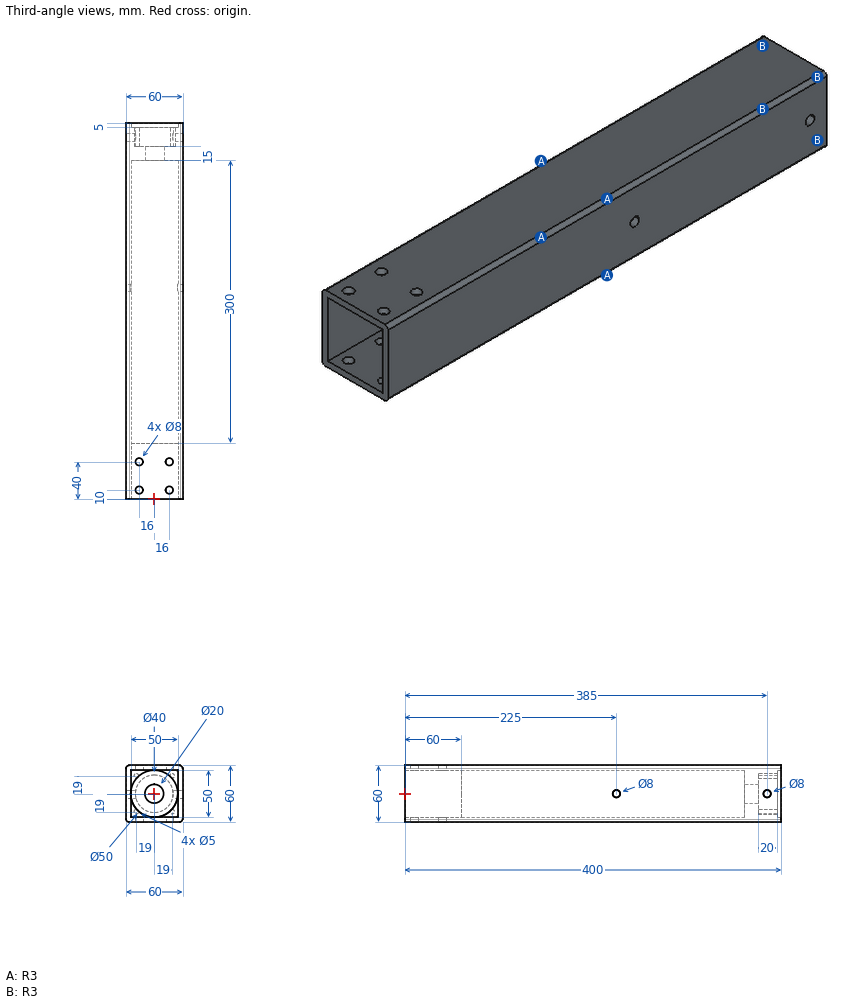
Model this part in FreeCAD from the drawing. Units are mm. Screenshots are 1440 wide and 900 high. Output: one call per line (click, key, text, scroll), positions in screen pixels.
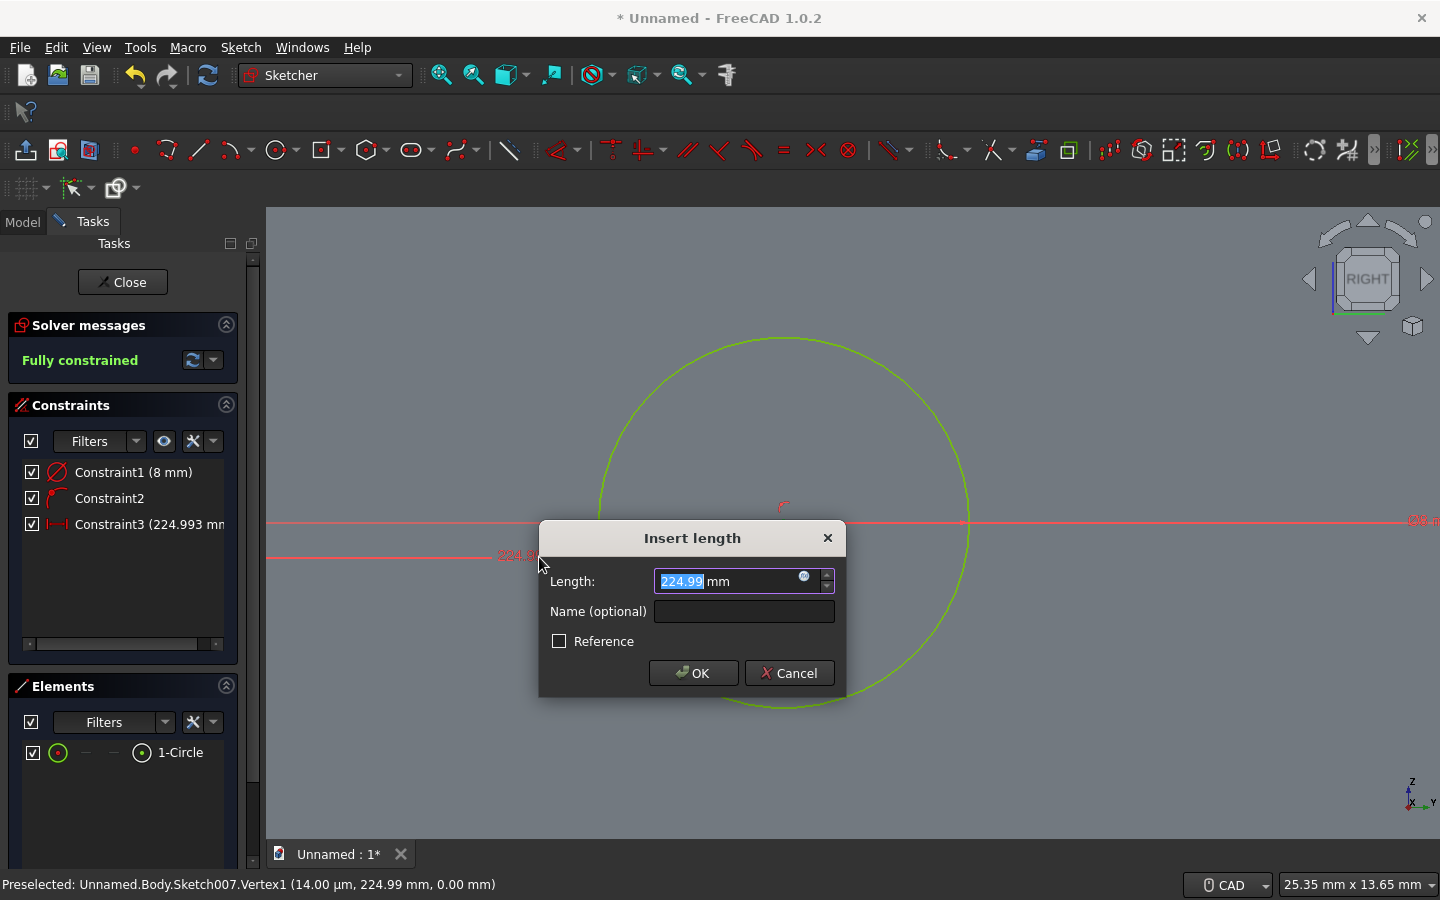
text(225)
key(Return)
key(Escape)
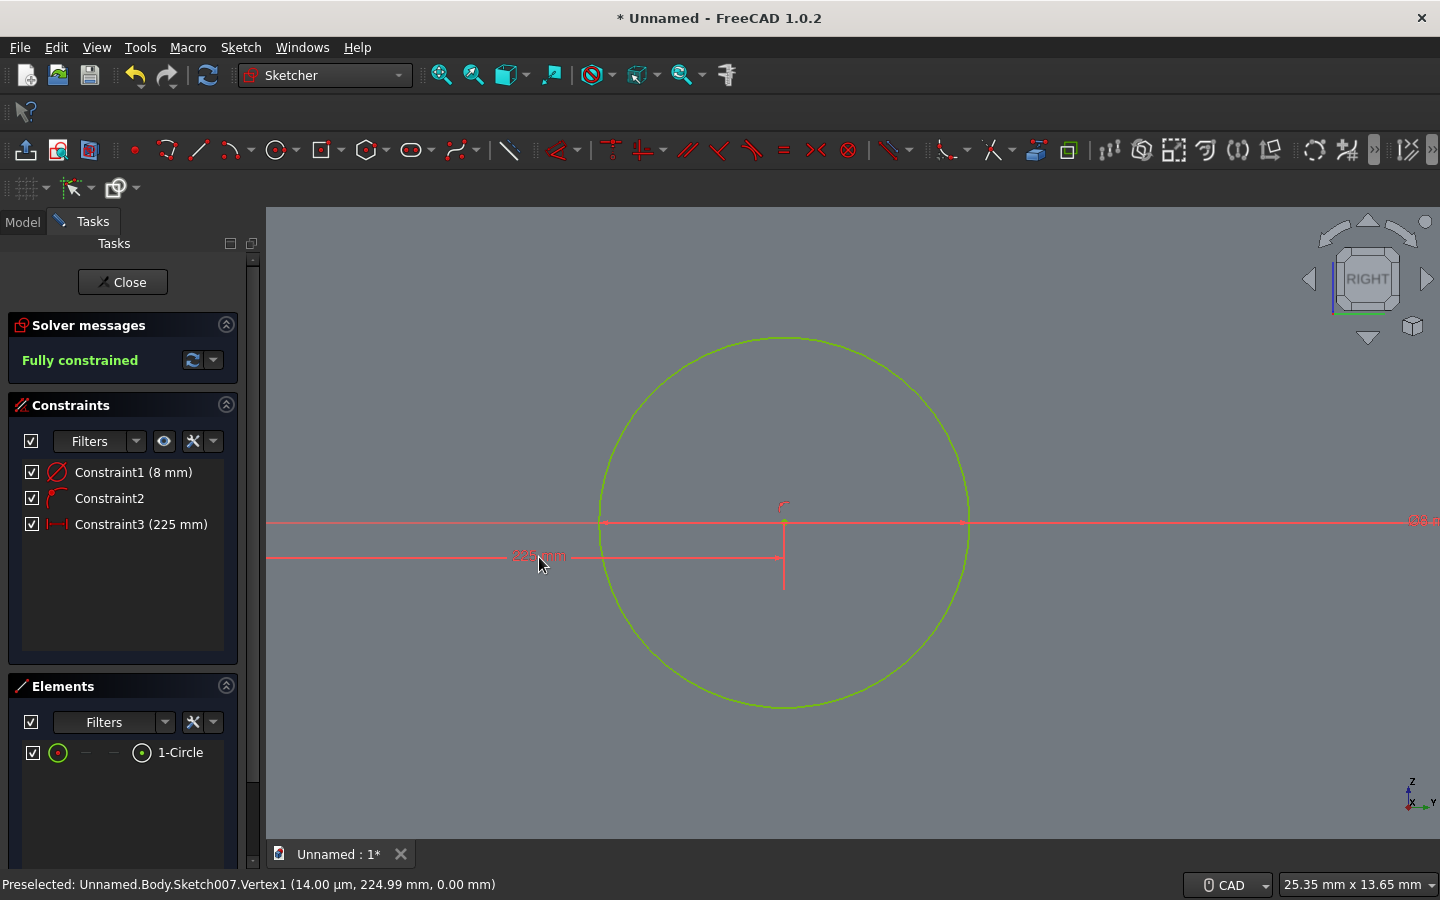
click(123, 282)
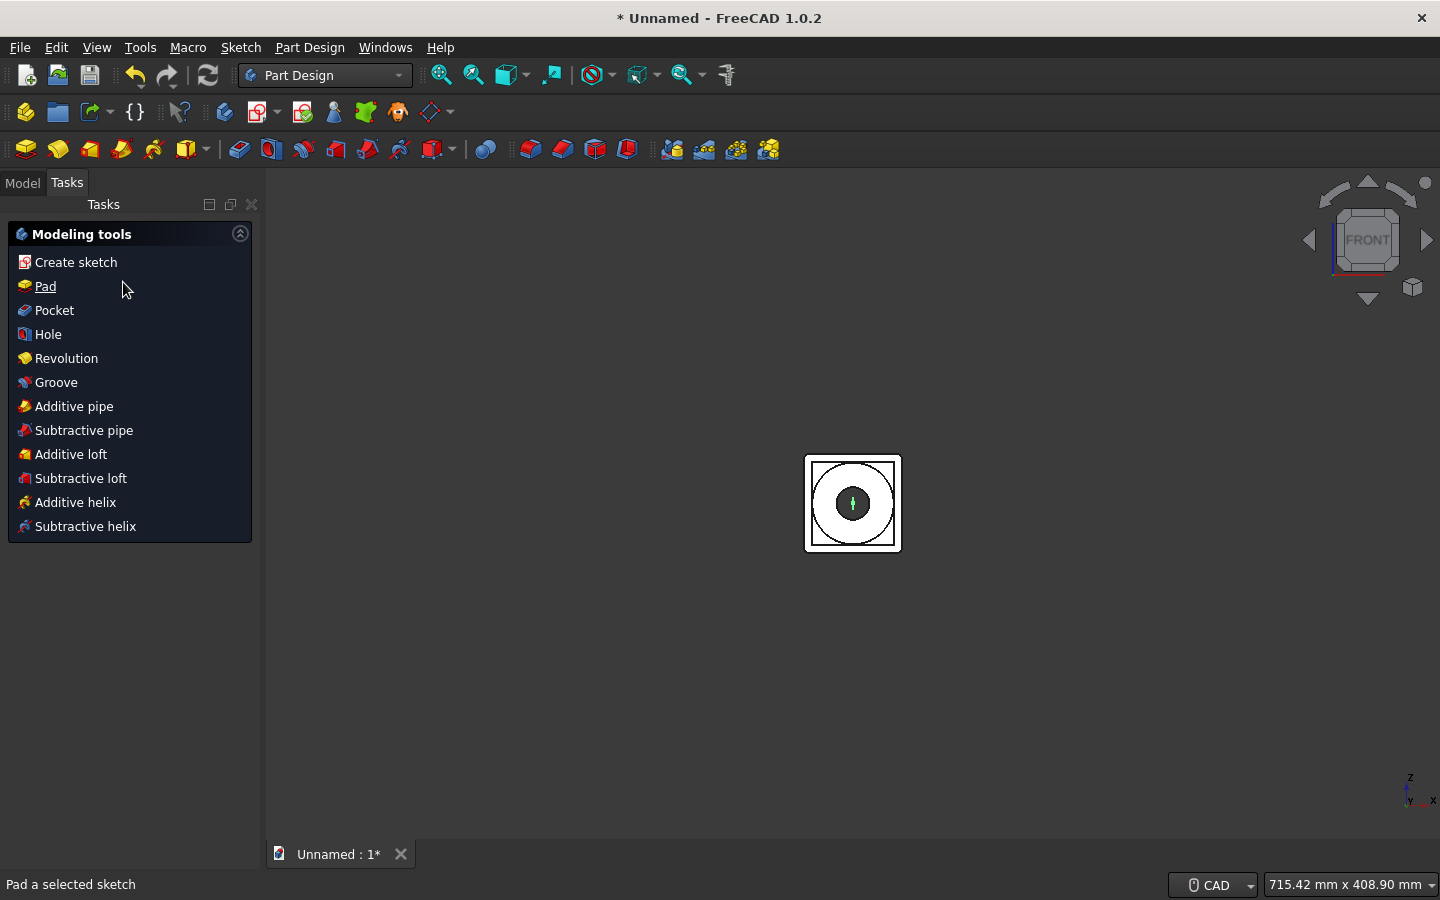
click(240, 150)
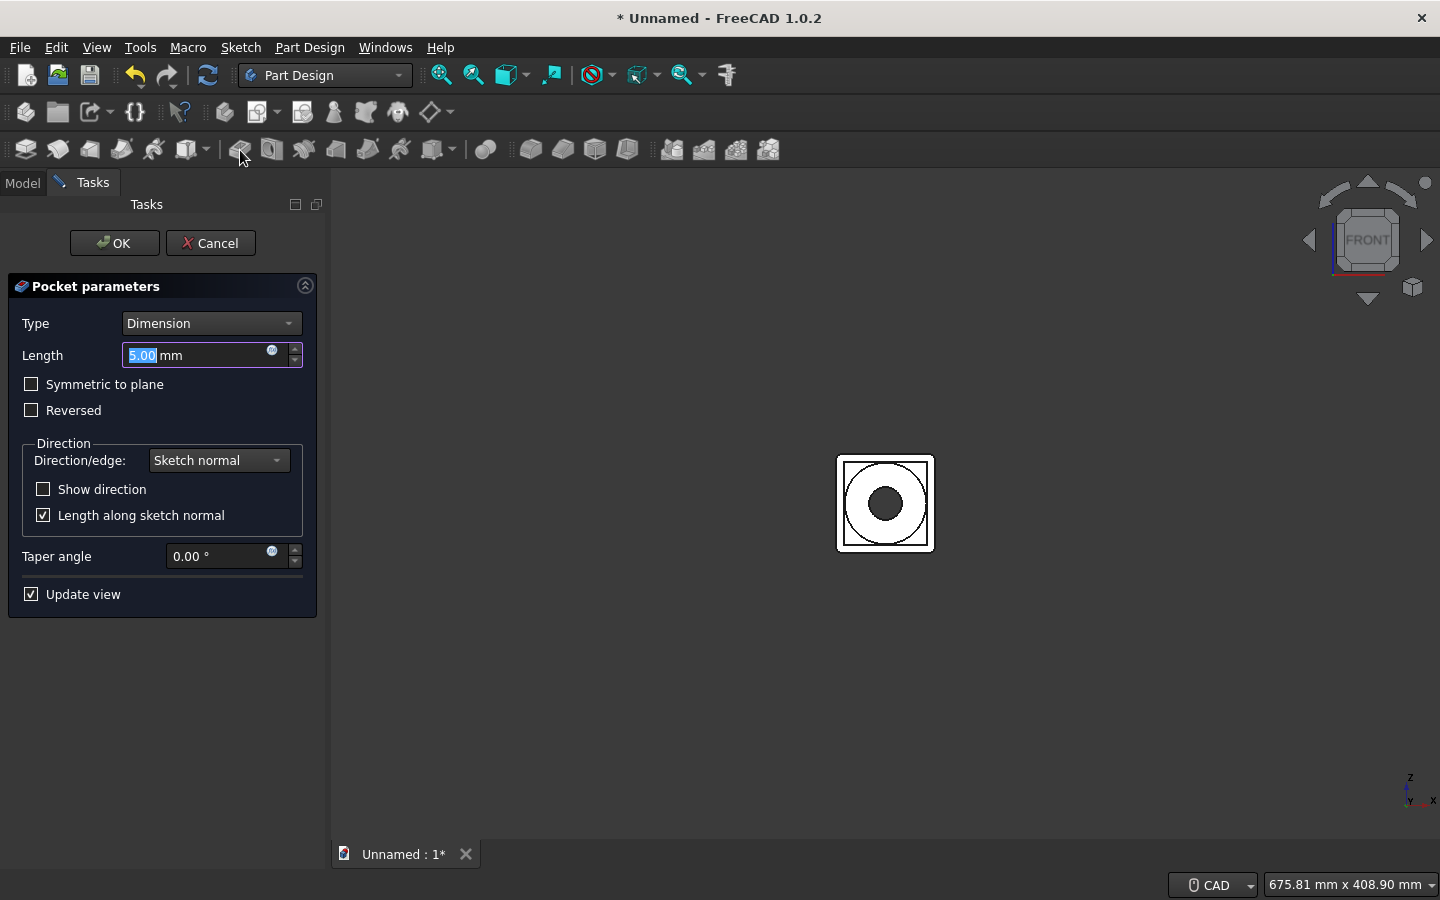
text(60)
key(Tab)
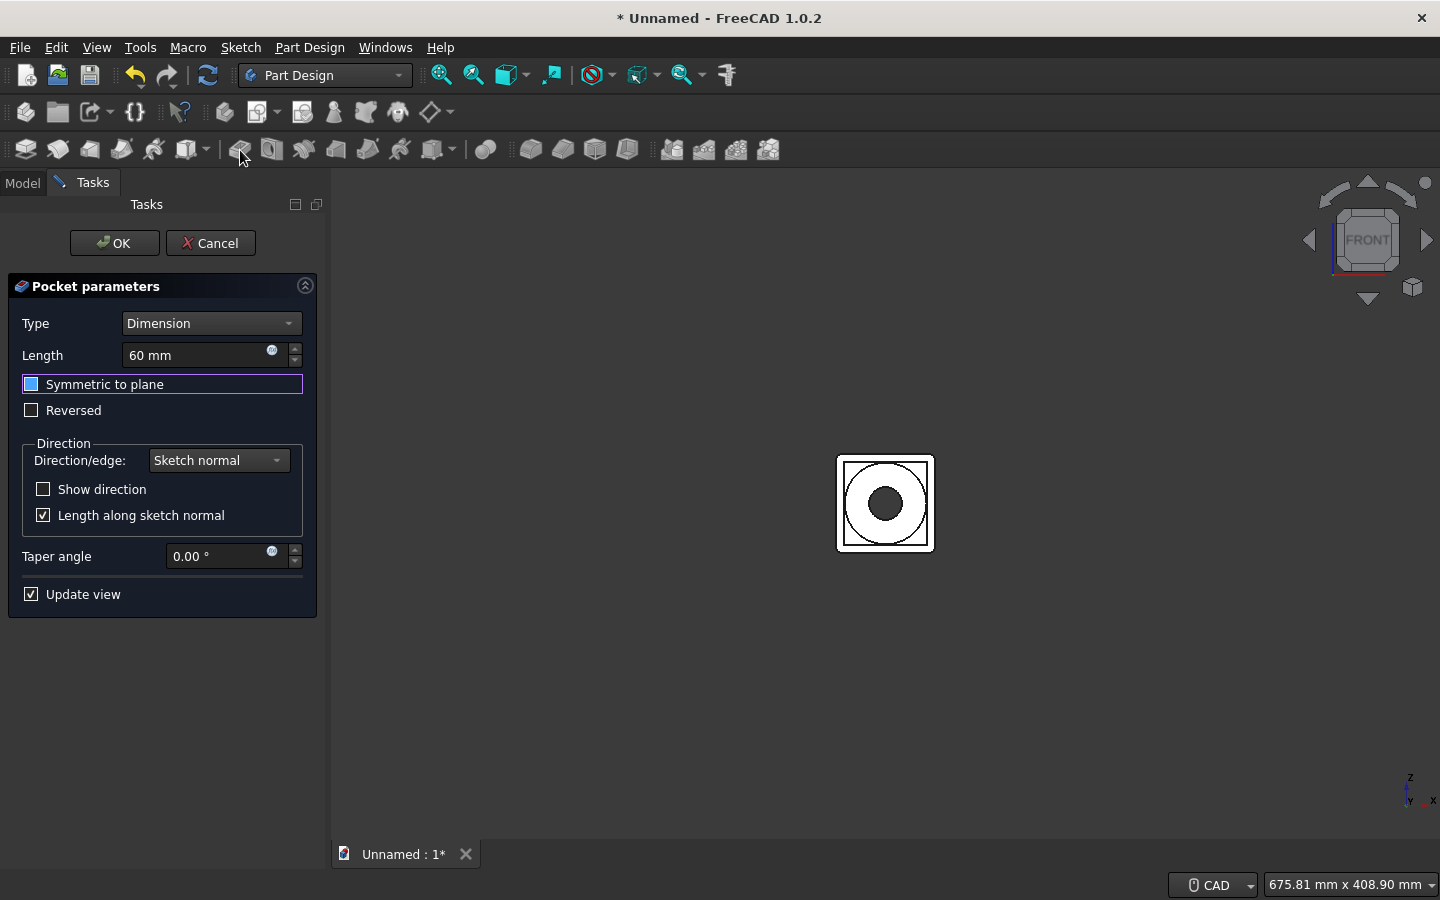
click(30, 384)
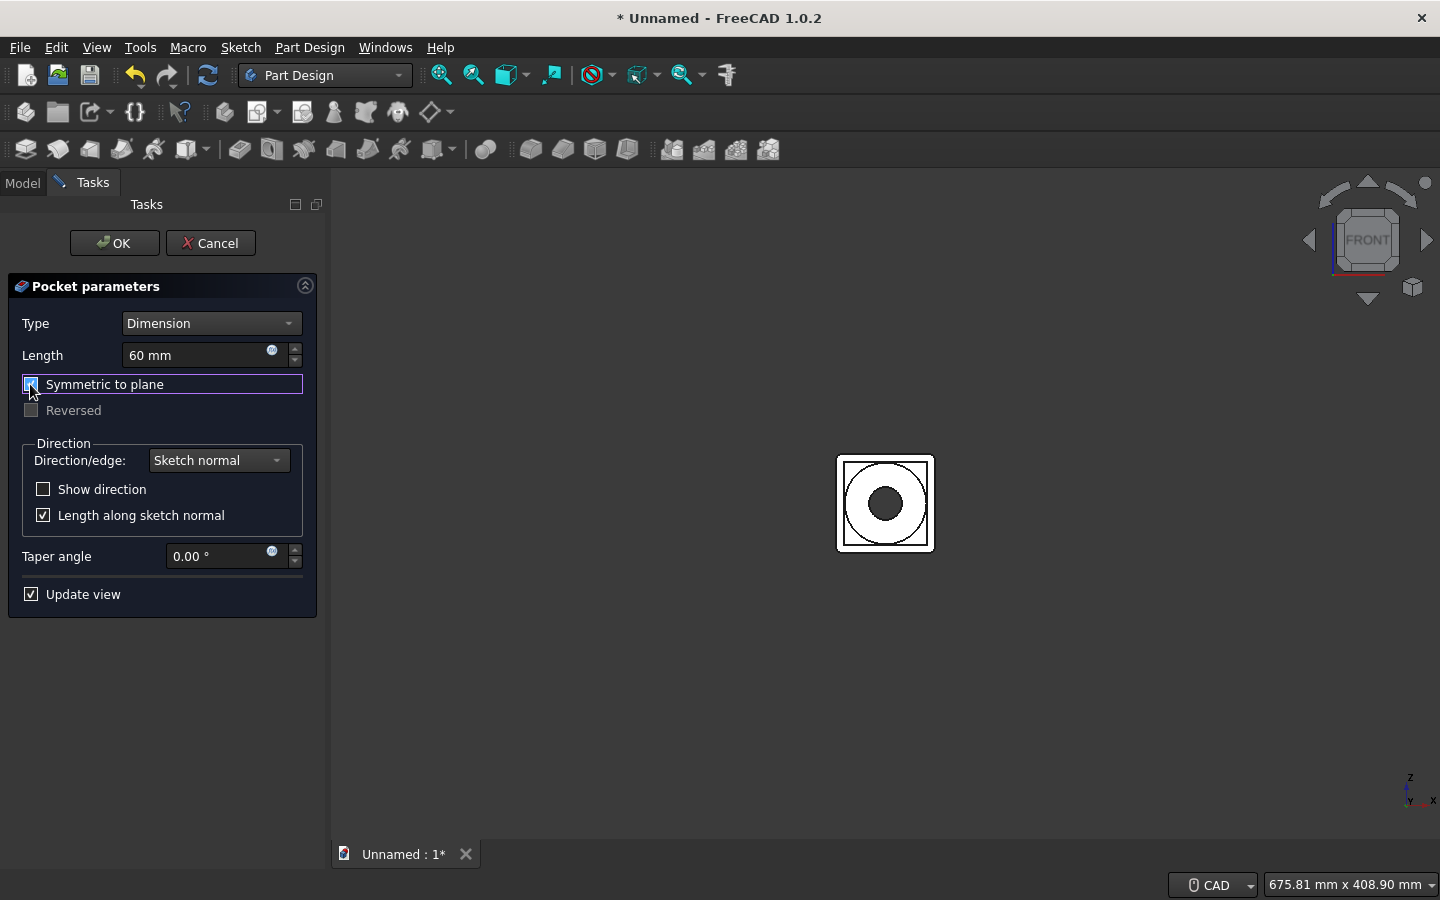
click(115, 243)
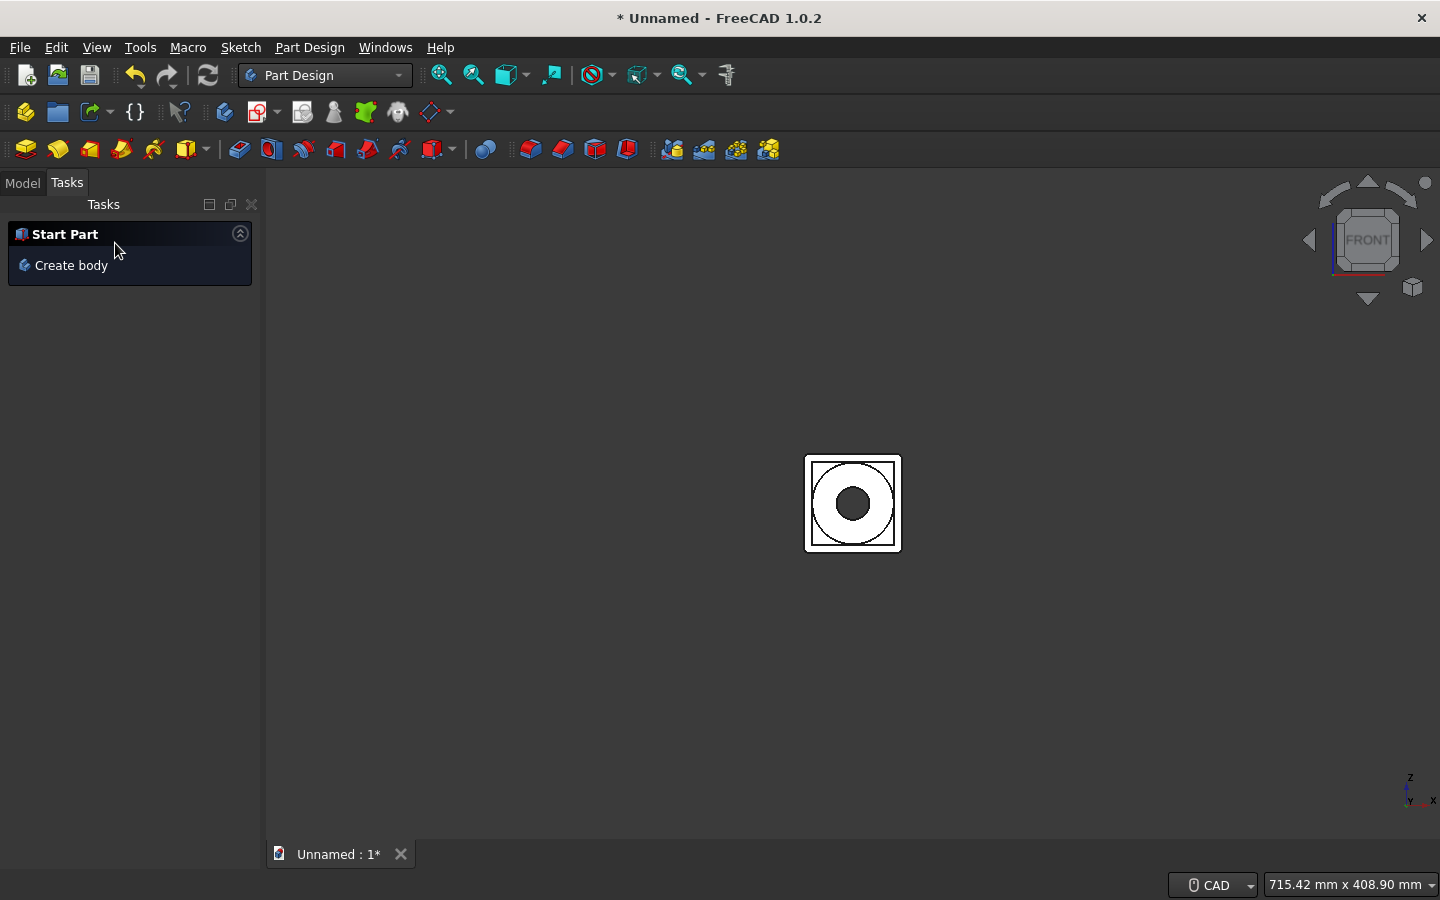
click(442, 76)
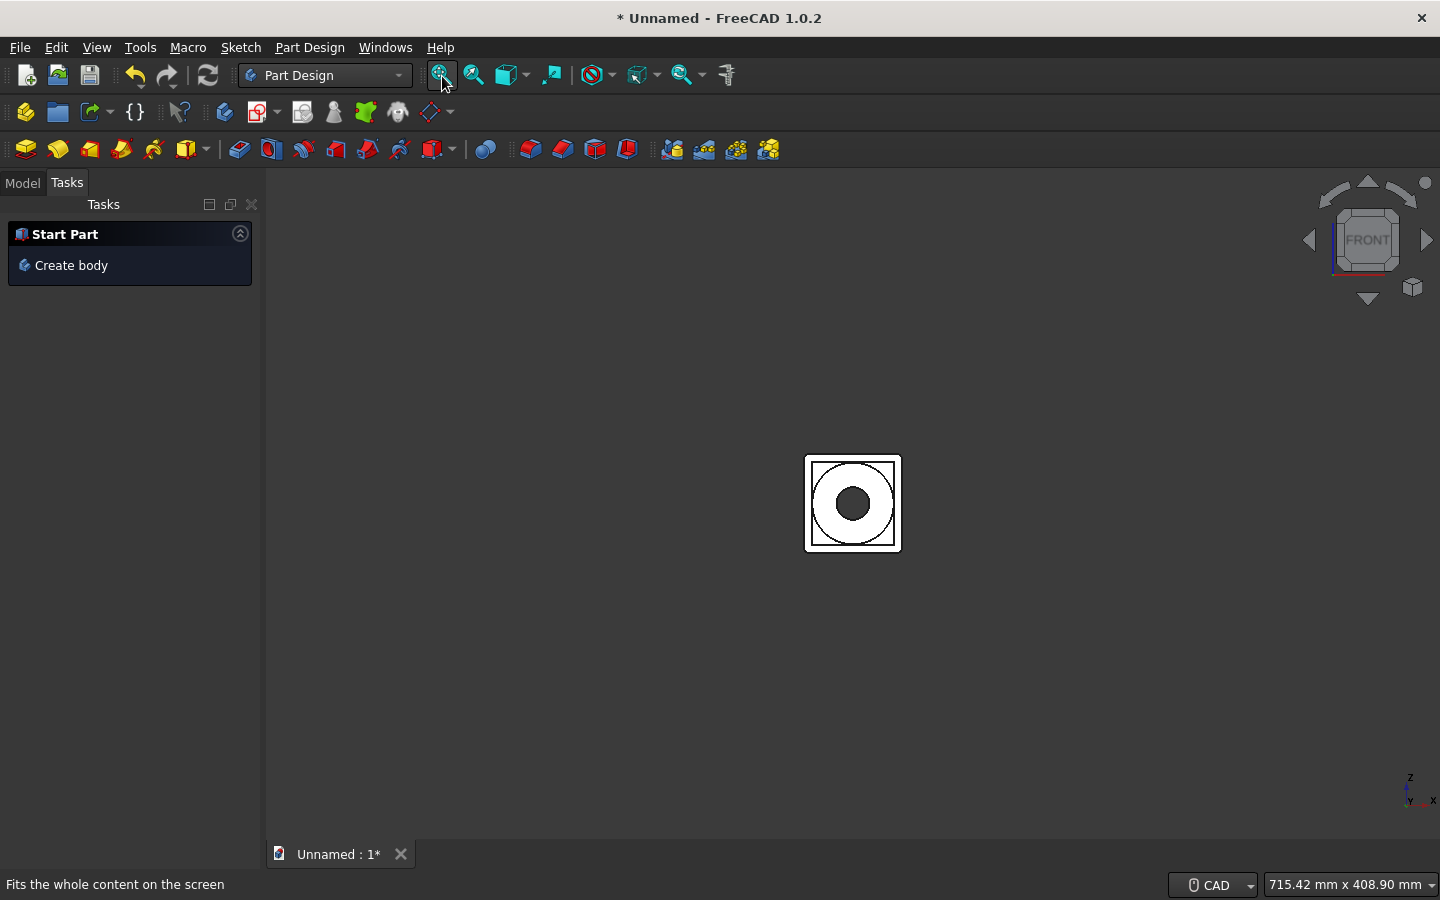
click(258, 112)